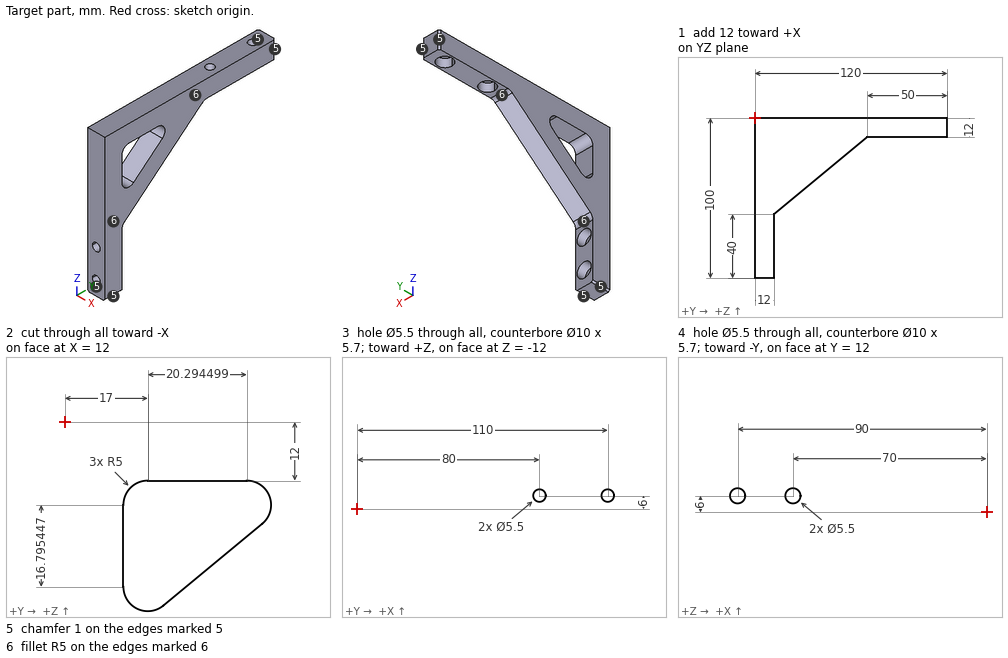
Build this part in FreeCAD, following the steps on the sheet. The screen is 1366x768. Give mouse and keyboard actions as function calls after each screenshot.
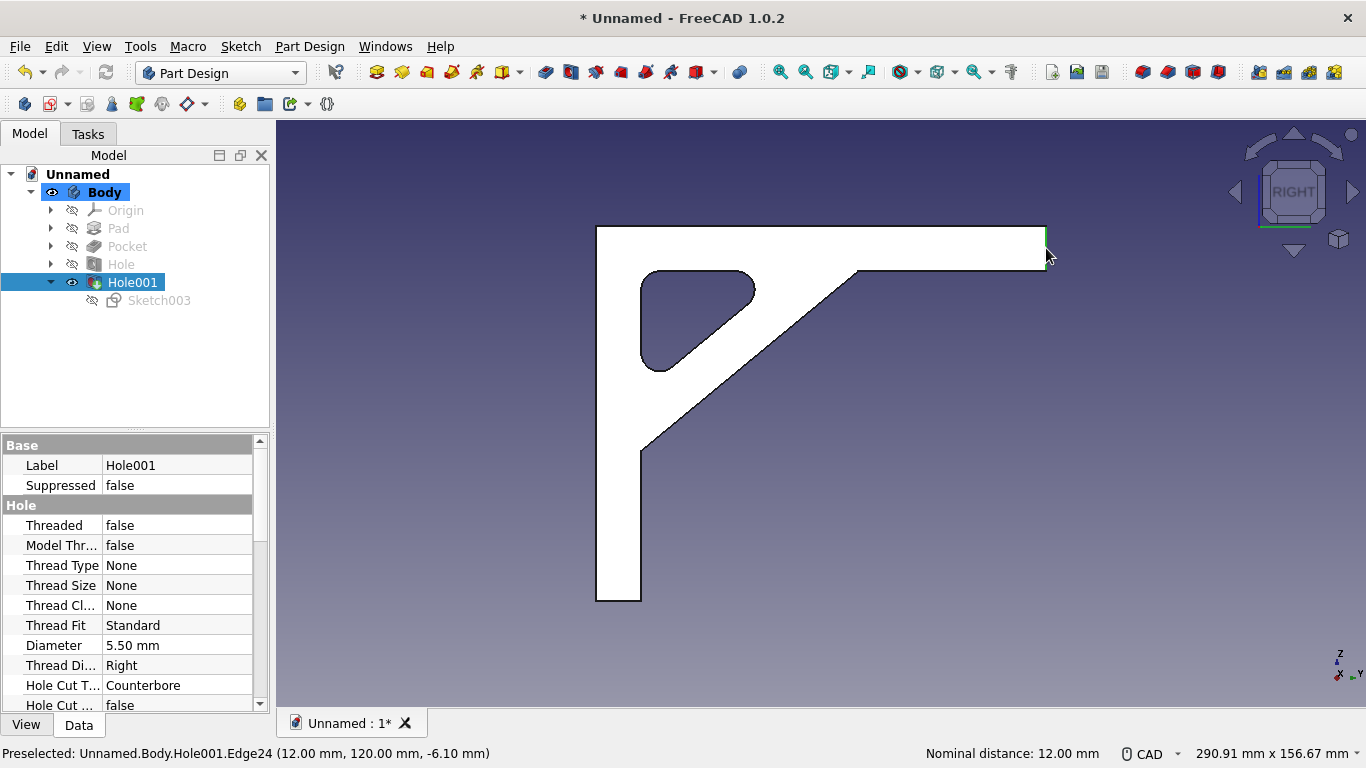
click(619, 600, ctrl)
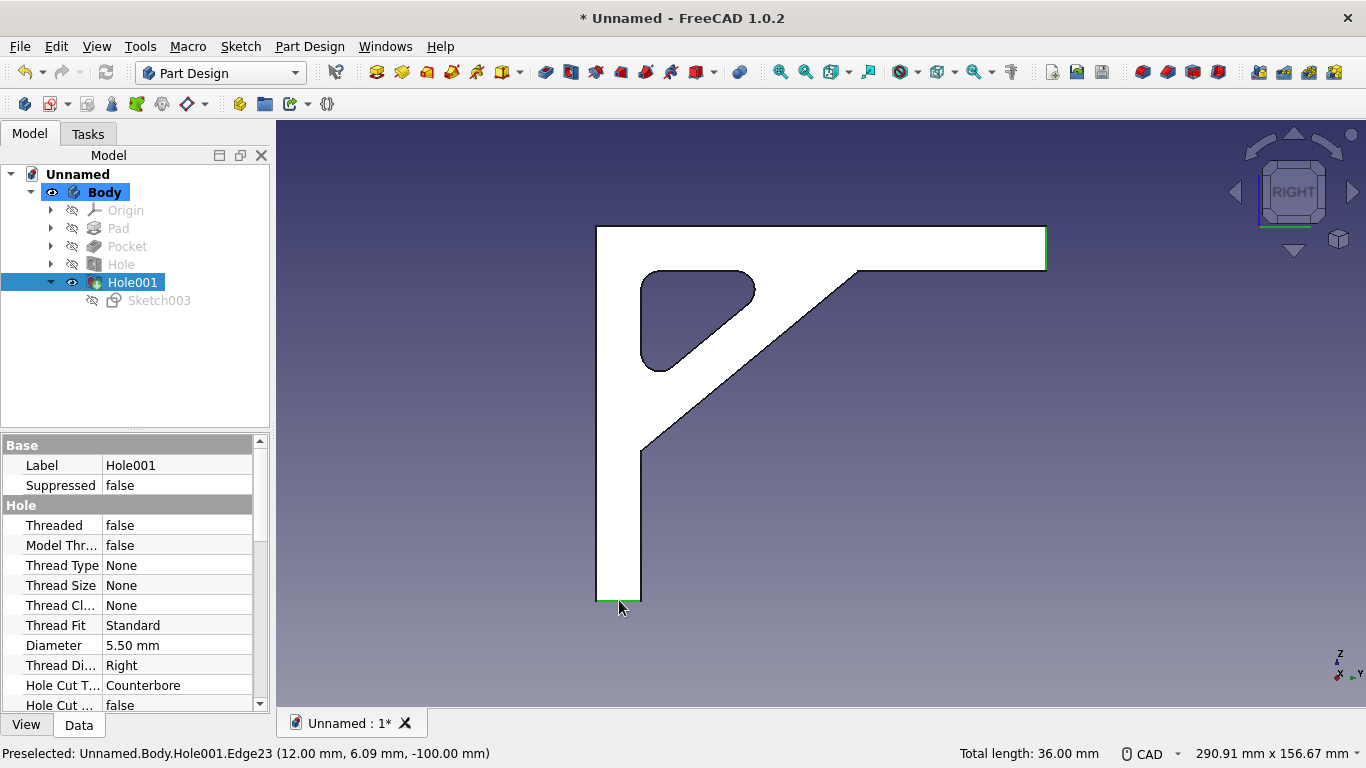
key(5)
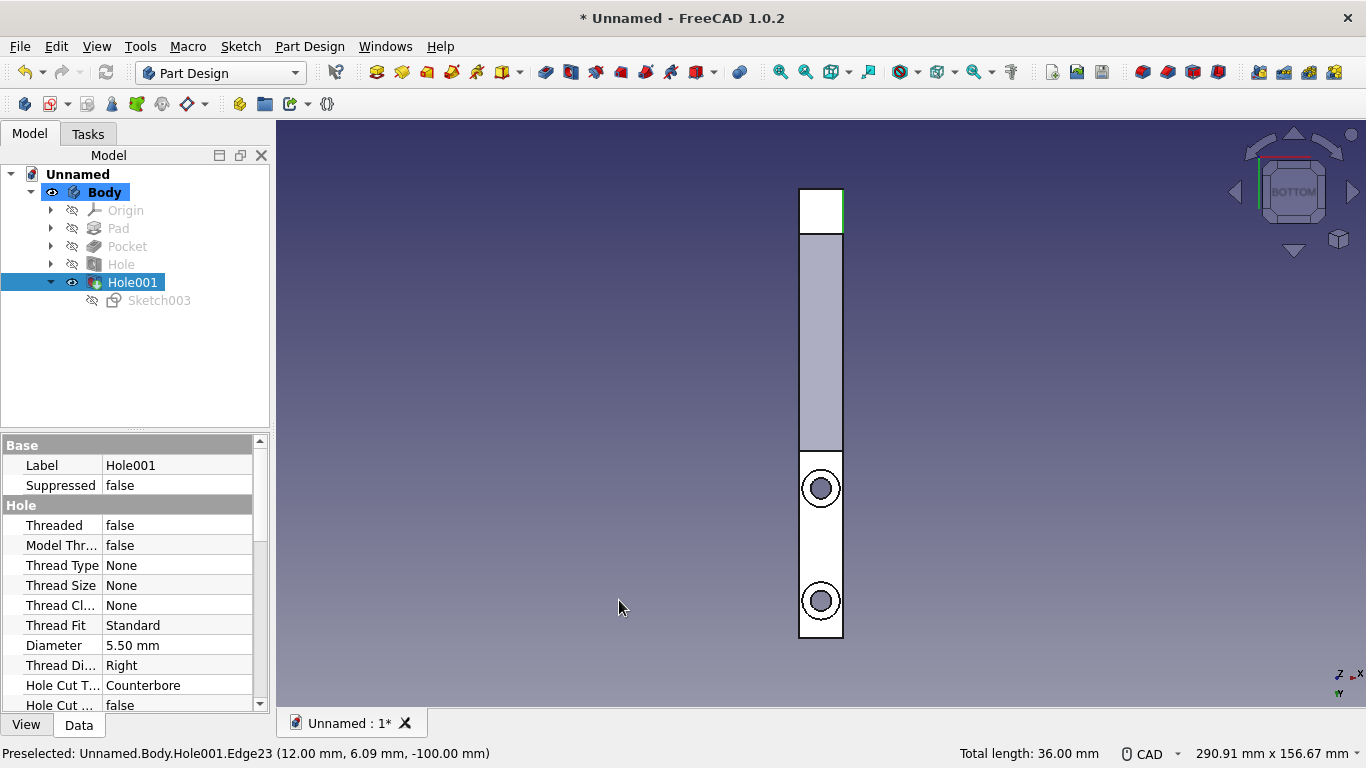
click(799, 210, ctrl)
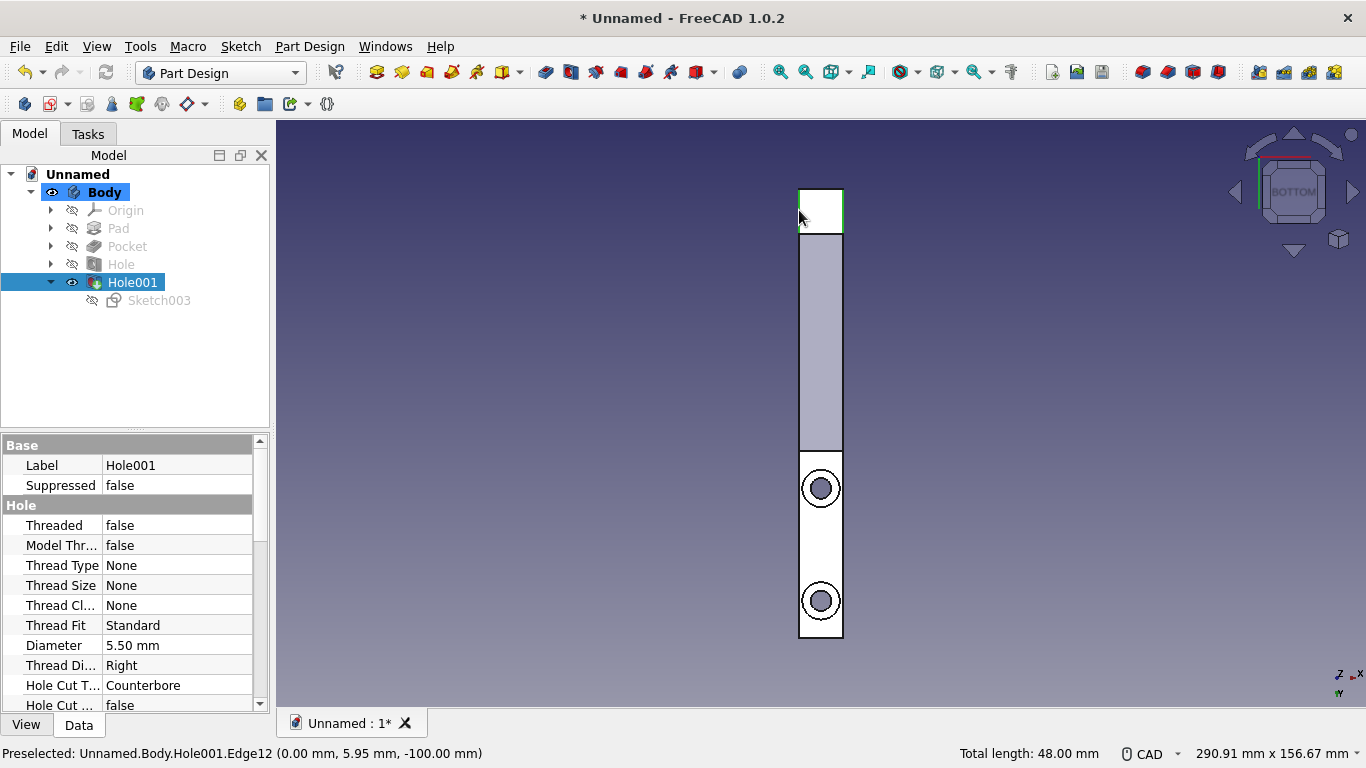
click(1168, 72)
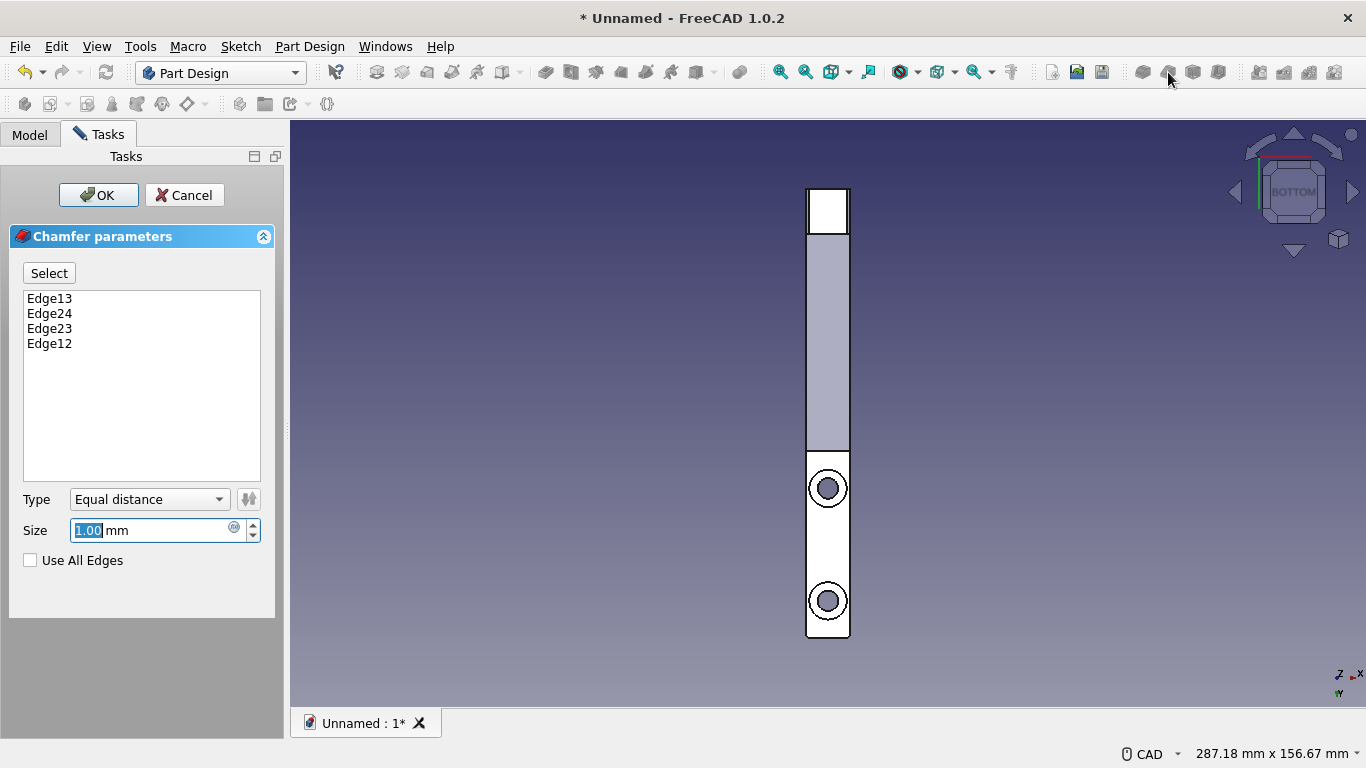
text(1)
key(Tab)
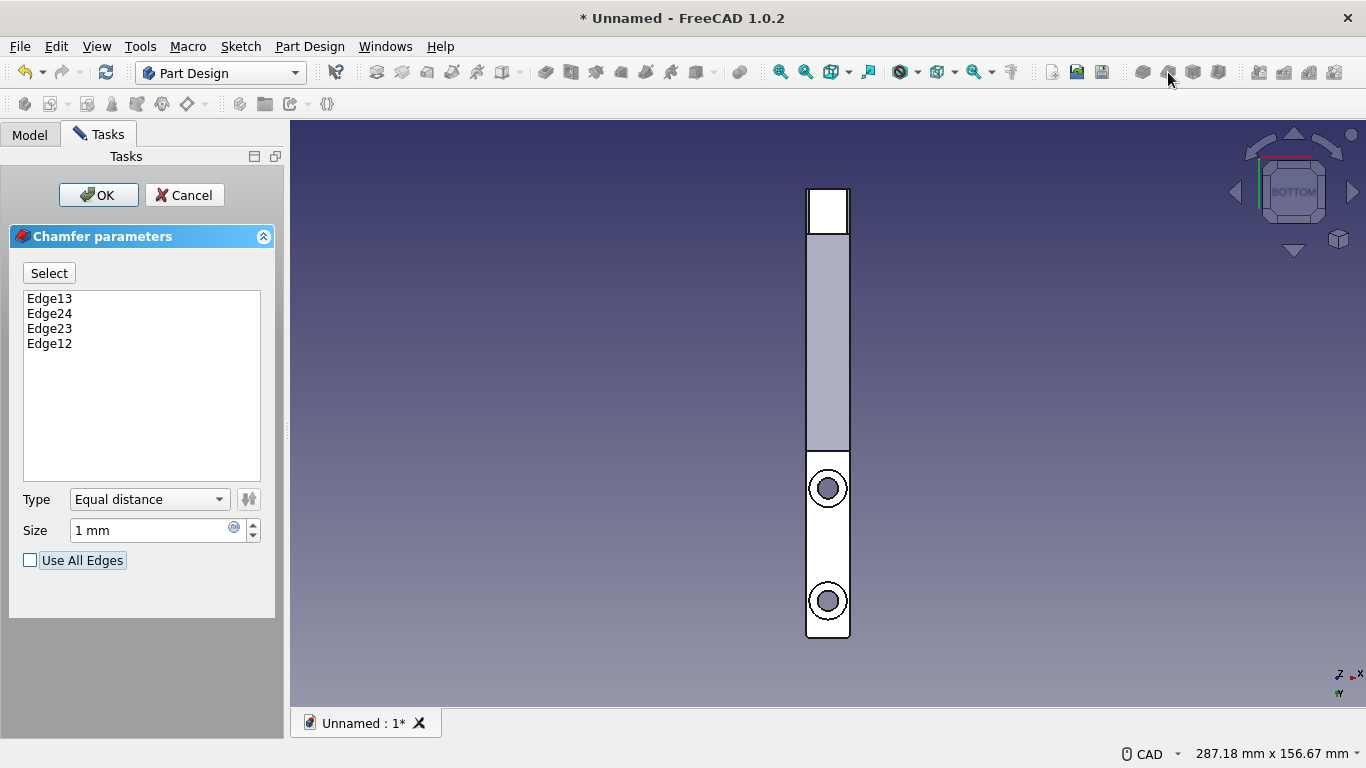
click(99, 195)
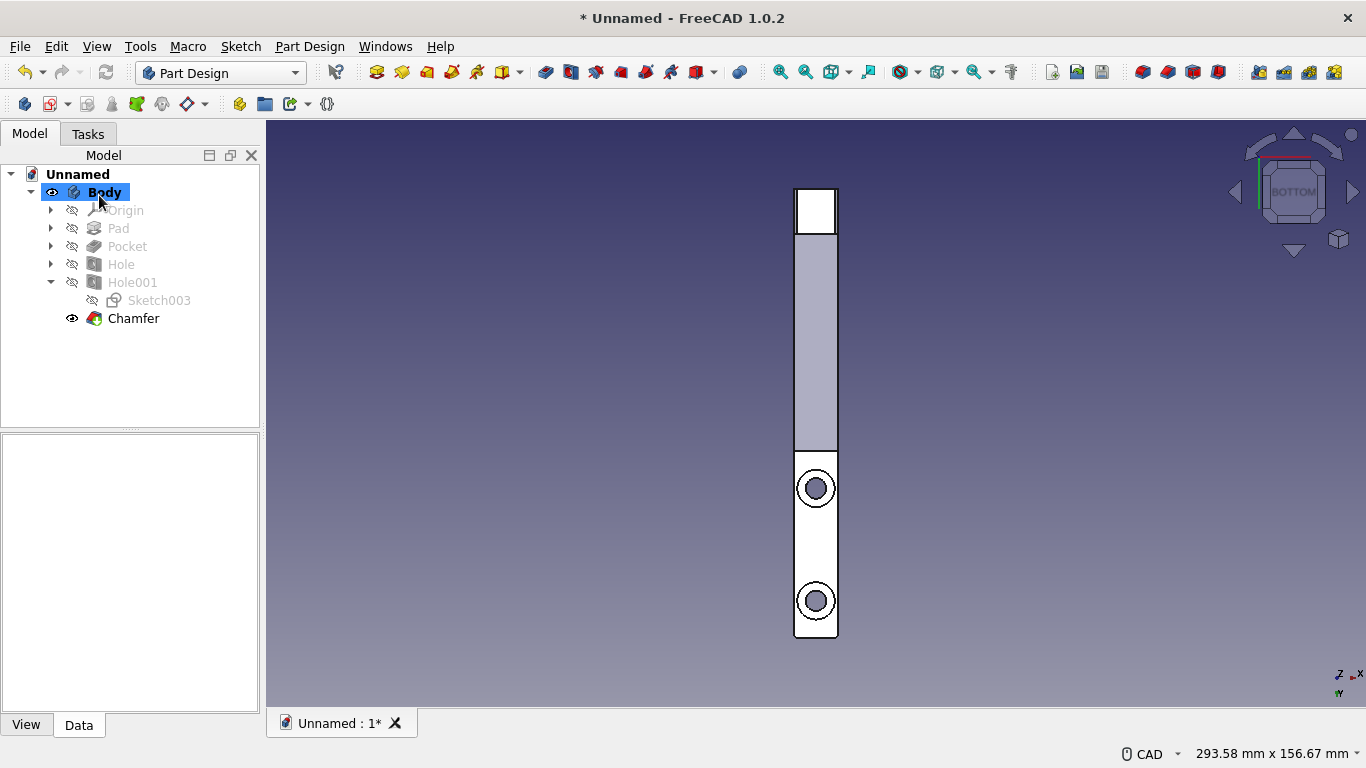
key(0)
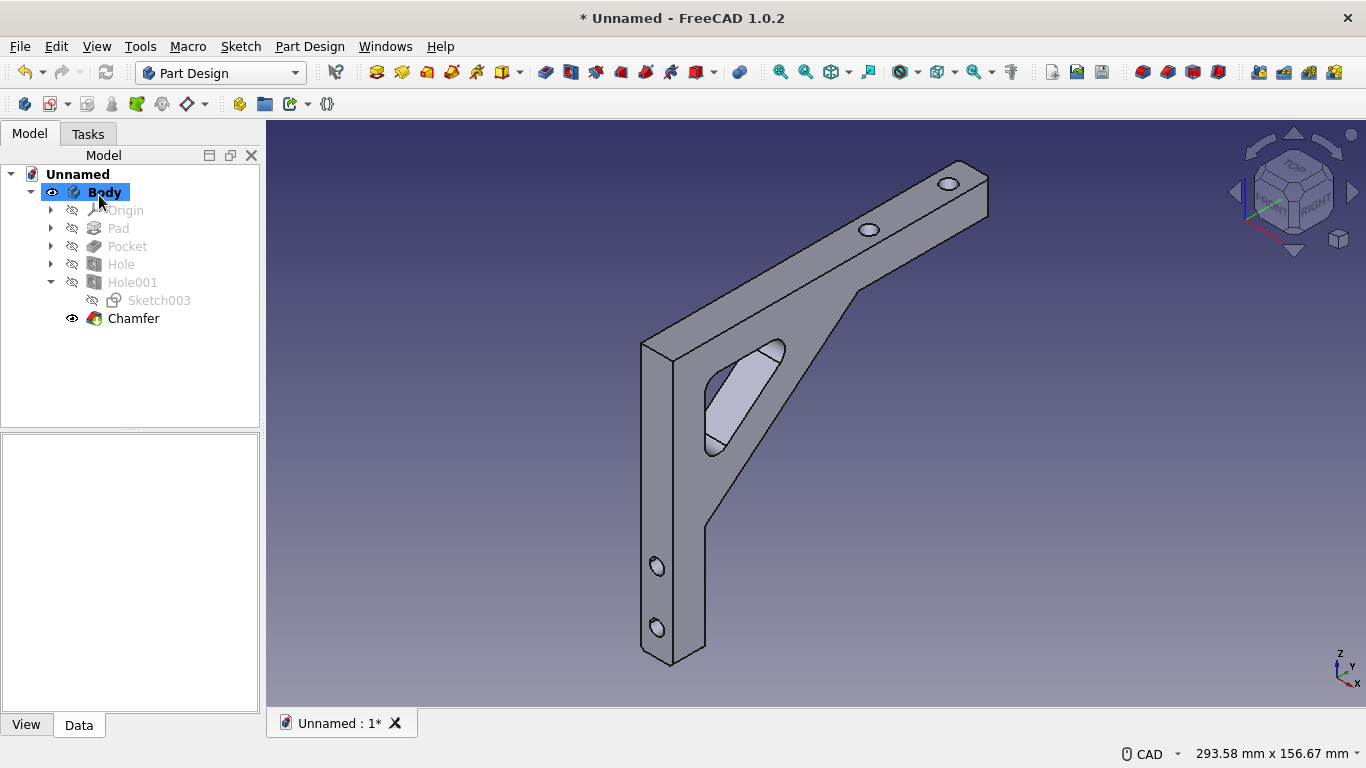
key(2)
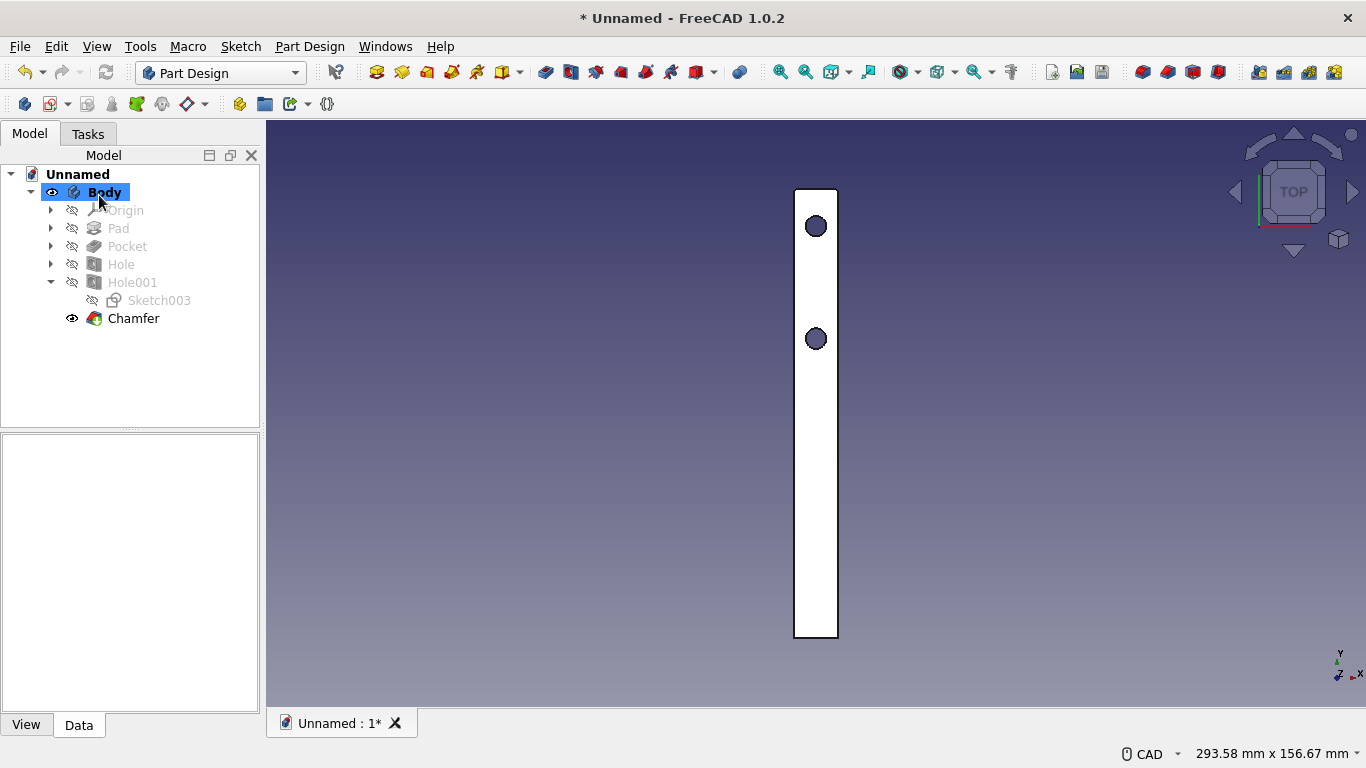
key(1)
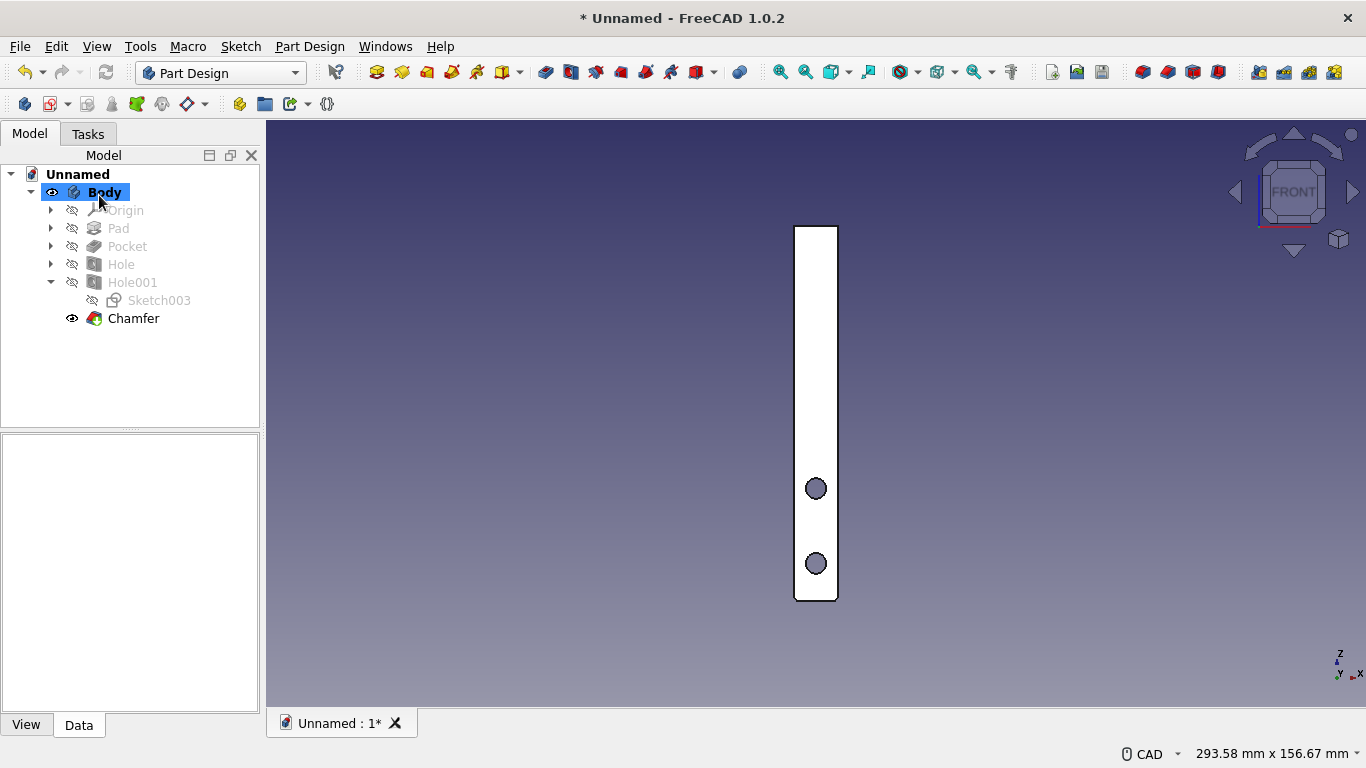
key(3)